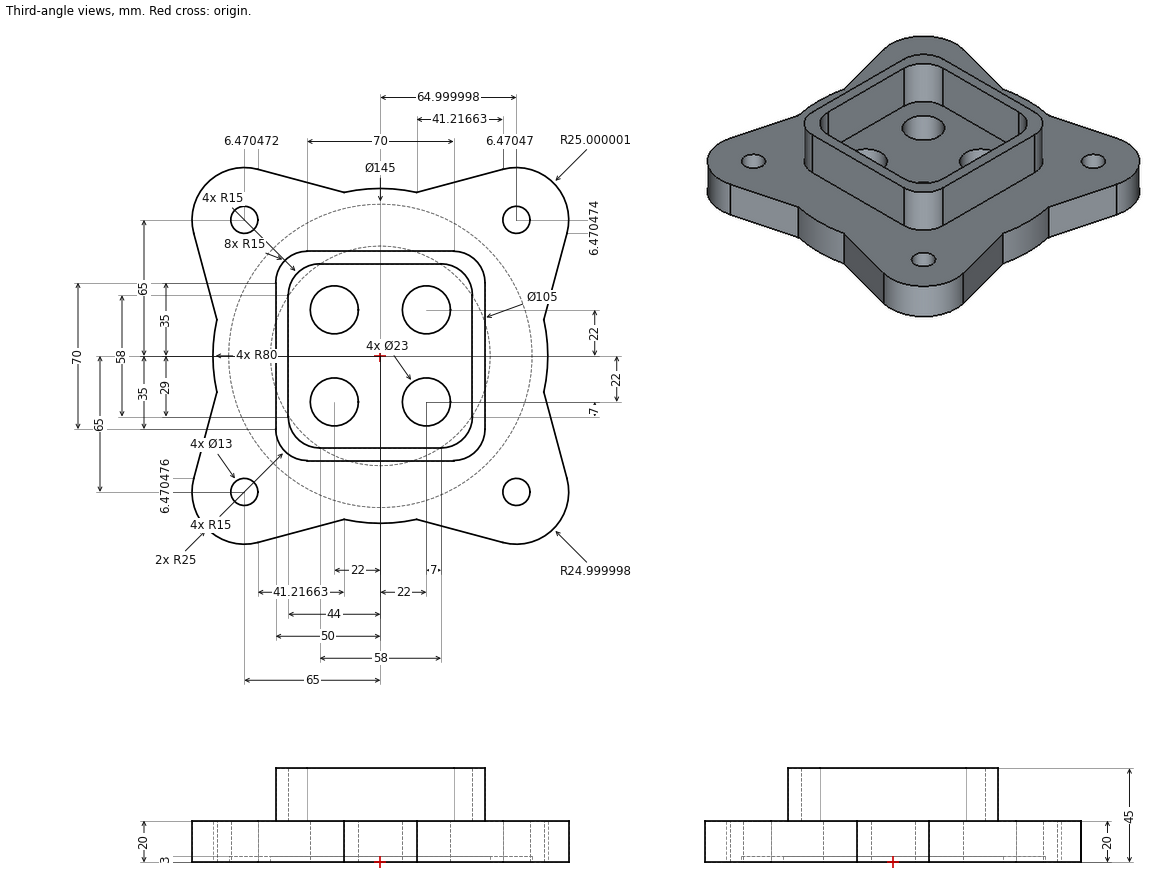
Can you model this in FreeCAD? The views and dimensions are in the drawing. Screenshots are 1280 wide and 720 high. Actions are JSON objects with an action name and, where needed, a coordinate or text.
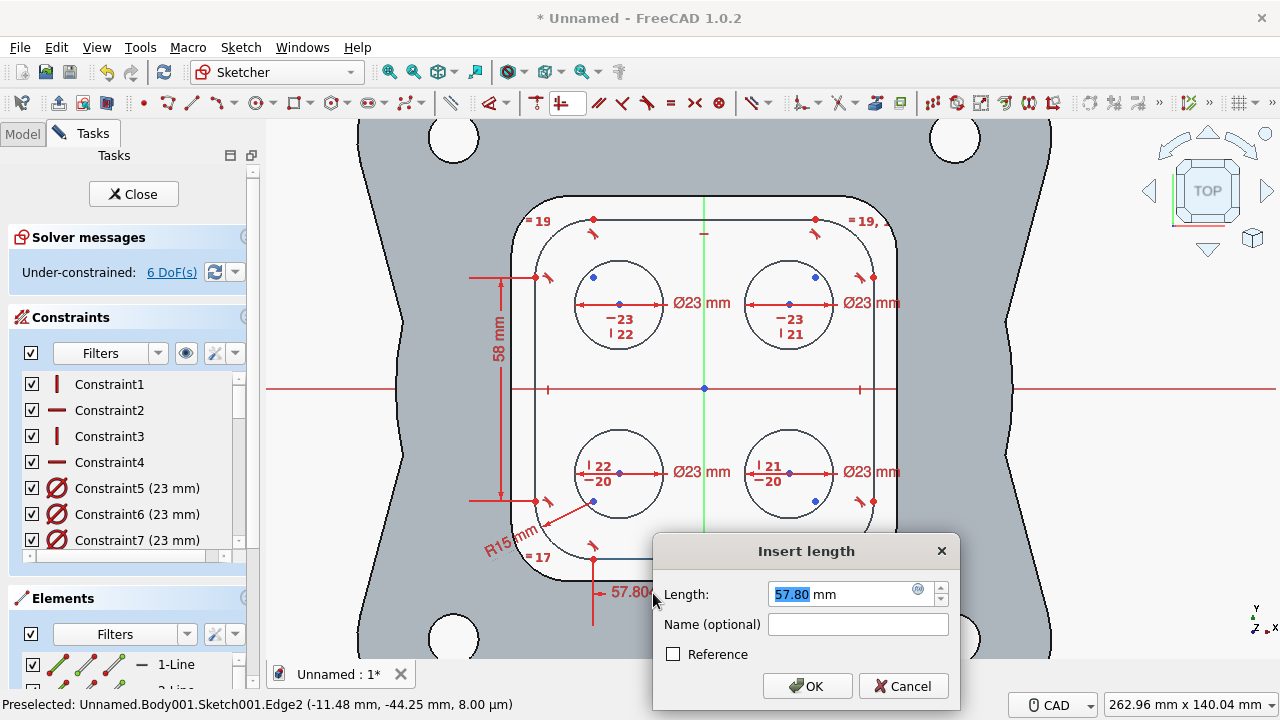
{"action": "type", "text": "58"}
{"action": "key", "text": "Return"}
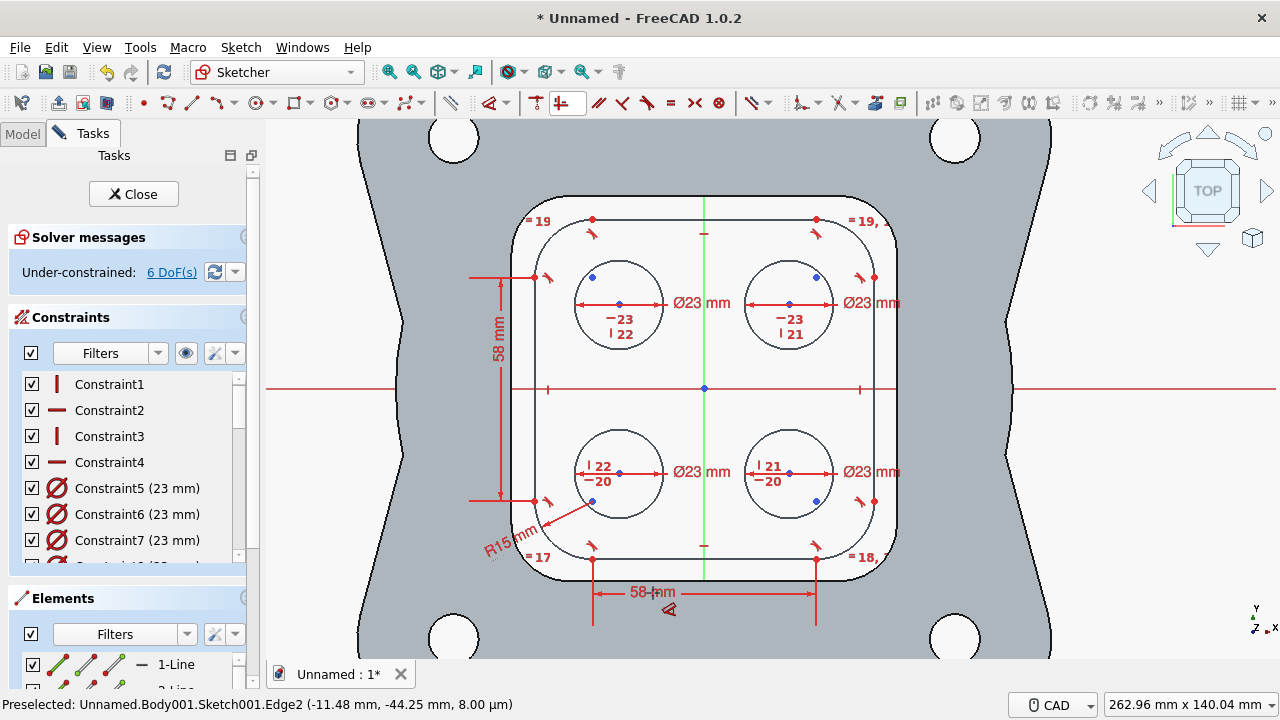
{"action": "left_click", "coordinate": [789, 474]}
{"action": "left_click", "coordinate": [727, 508]}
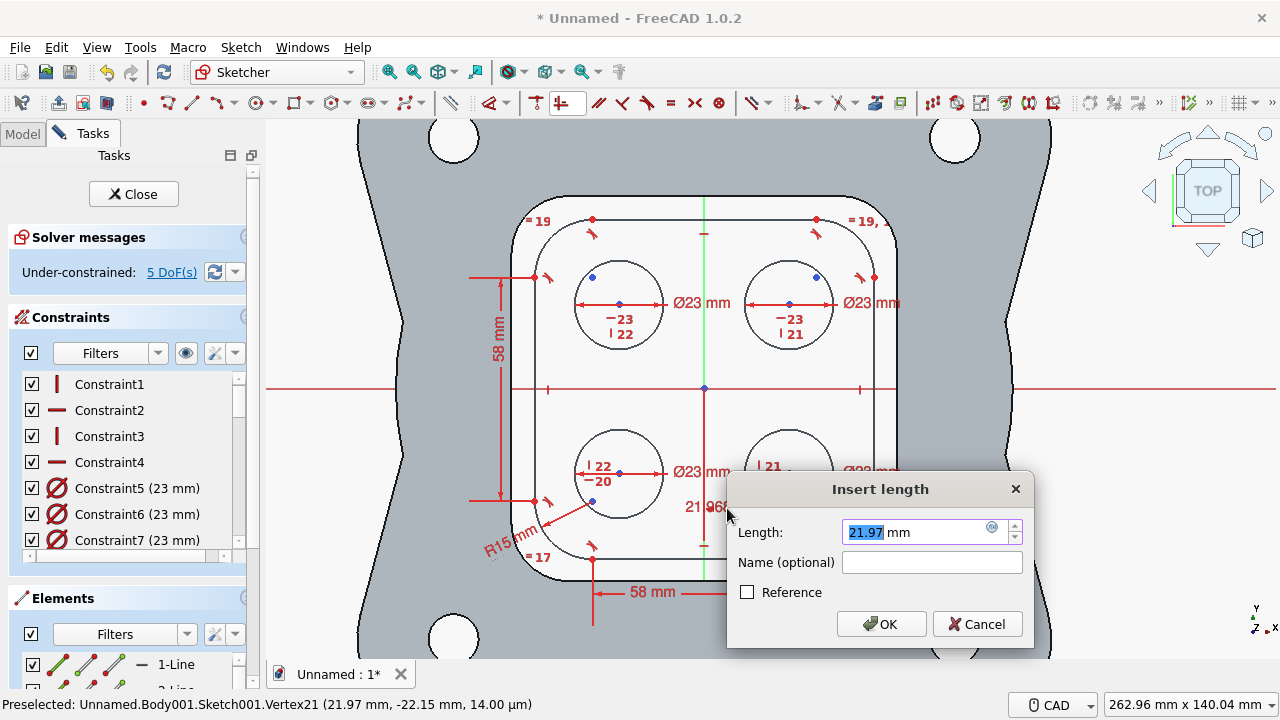
{"action": "type", "text": "22"}
{"action": "key", "text": "Return"}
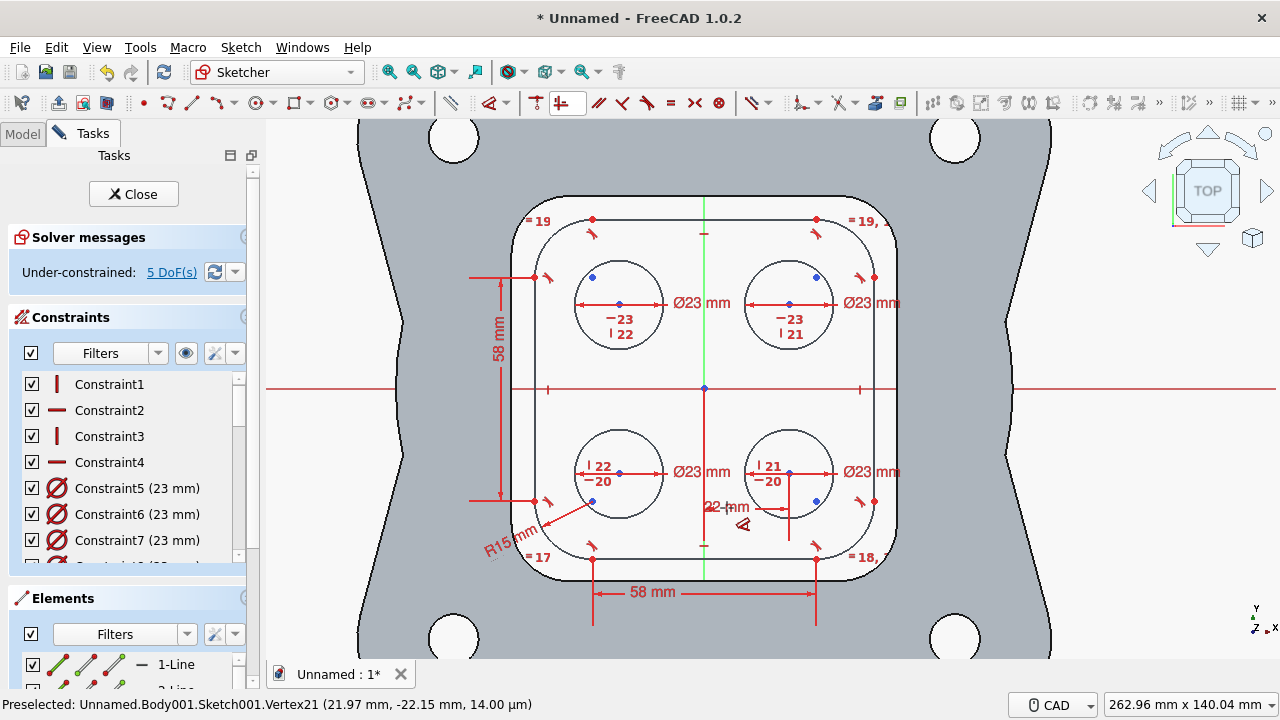
{"action": "left_click", "coordinate": [789, 474]}
{"action": "left_click", "coordinate": [823, 412]}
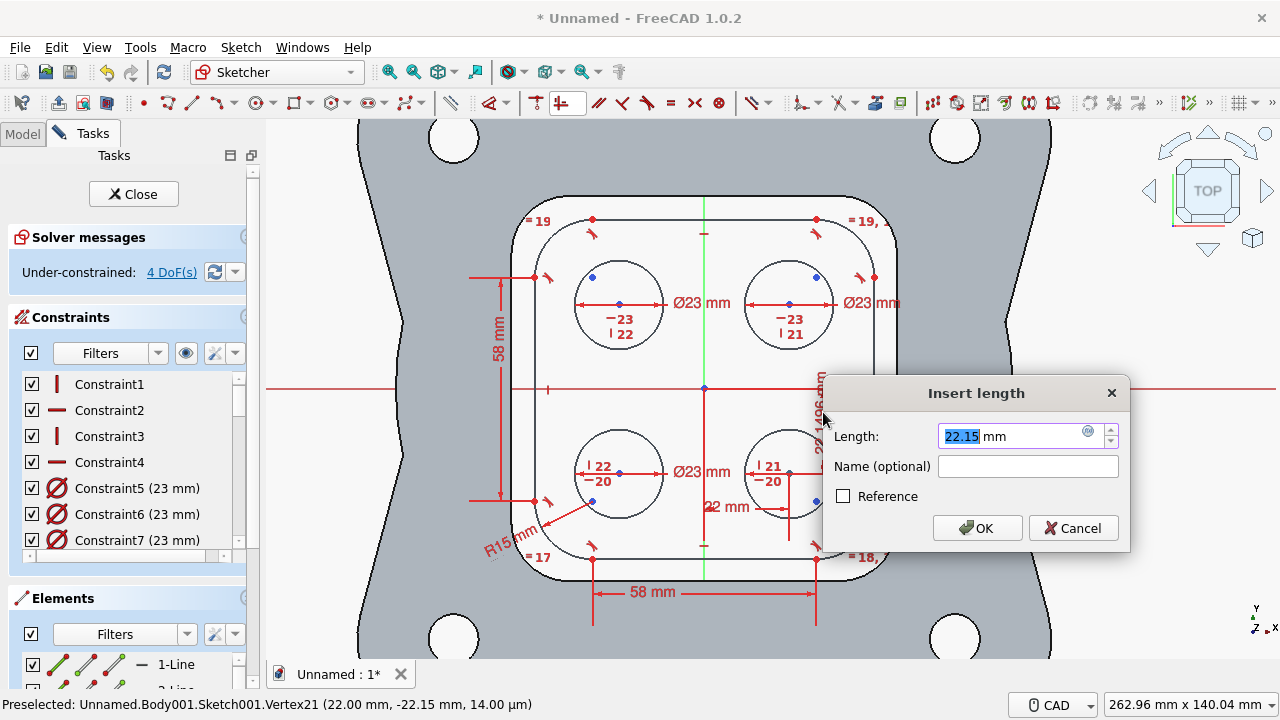
{"action": "type", "text": "22"}
{"action": "key", "text": "Return"}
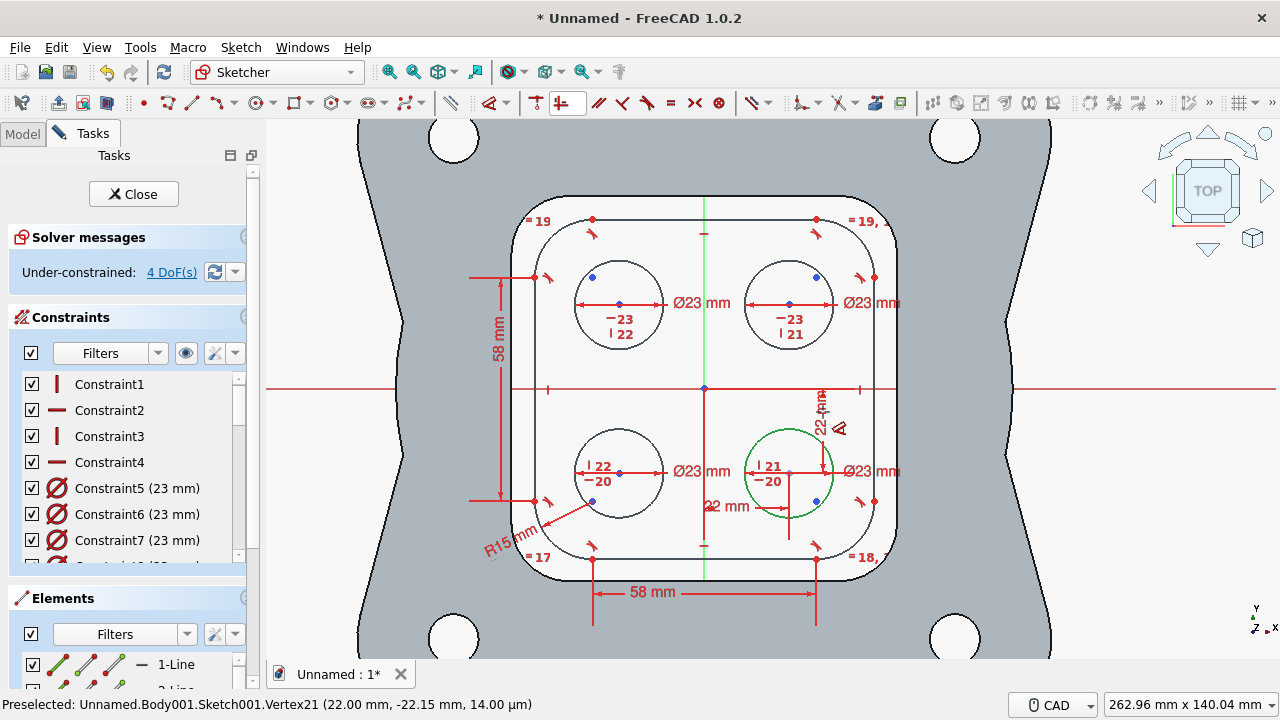
{"action": "left_click", "coordinate": [619, 473]}
{"action": "left_click", "coordinate": [662, 355]}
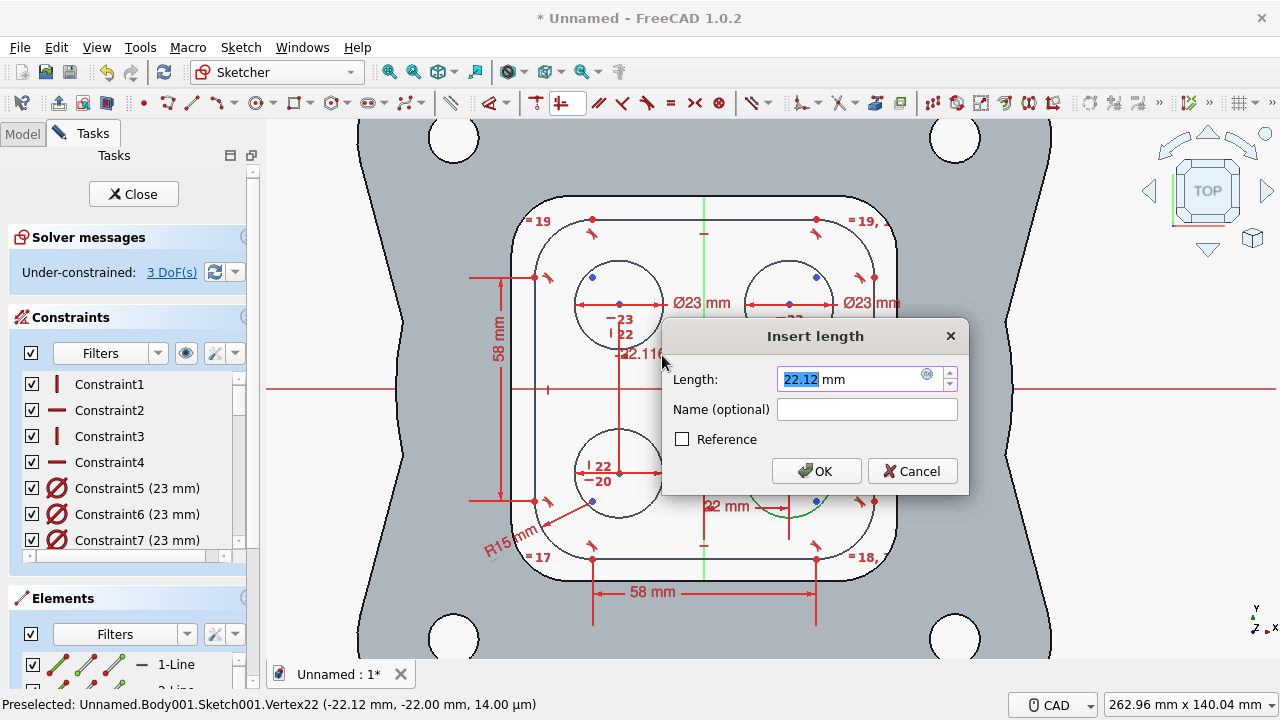
{"action": "type", "text": "22"}
{"action": "key", "text": "Return"}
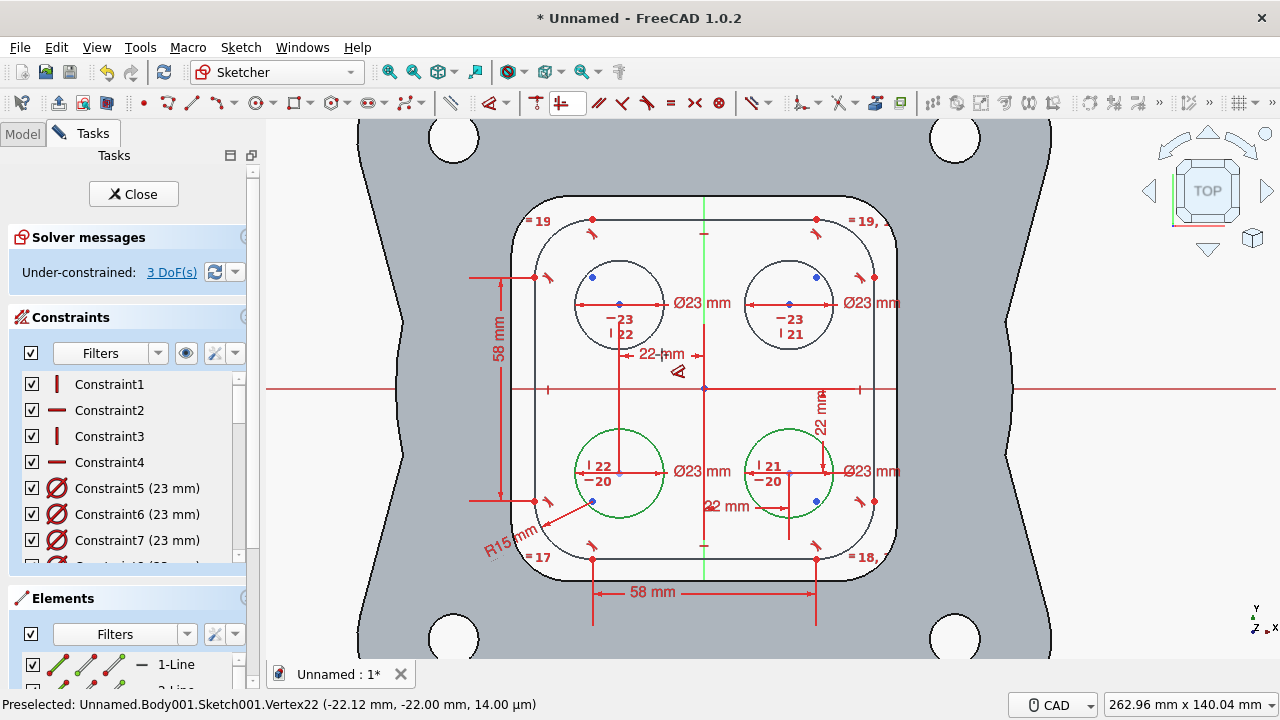
{"action": "left_click", "coordinate": [789, 305]}
{"action": "left_click", "coordinate": [823, 366]}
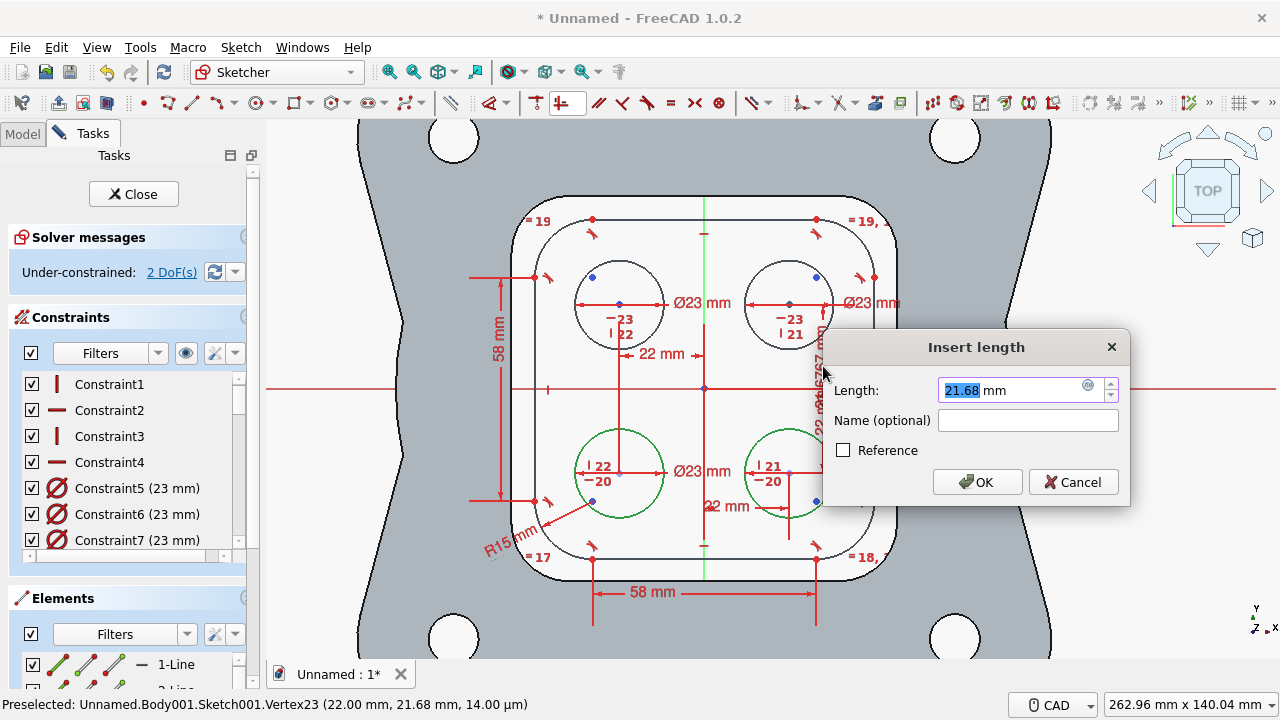
{"action": "type", "text": "22"}
{"action": "key", "text": "Return"}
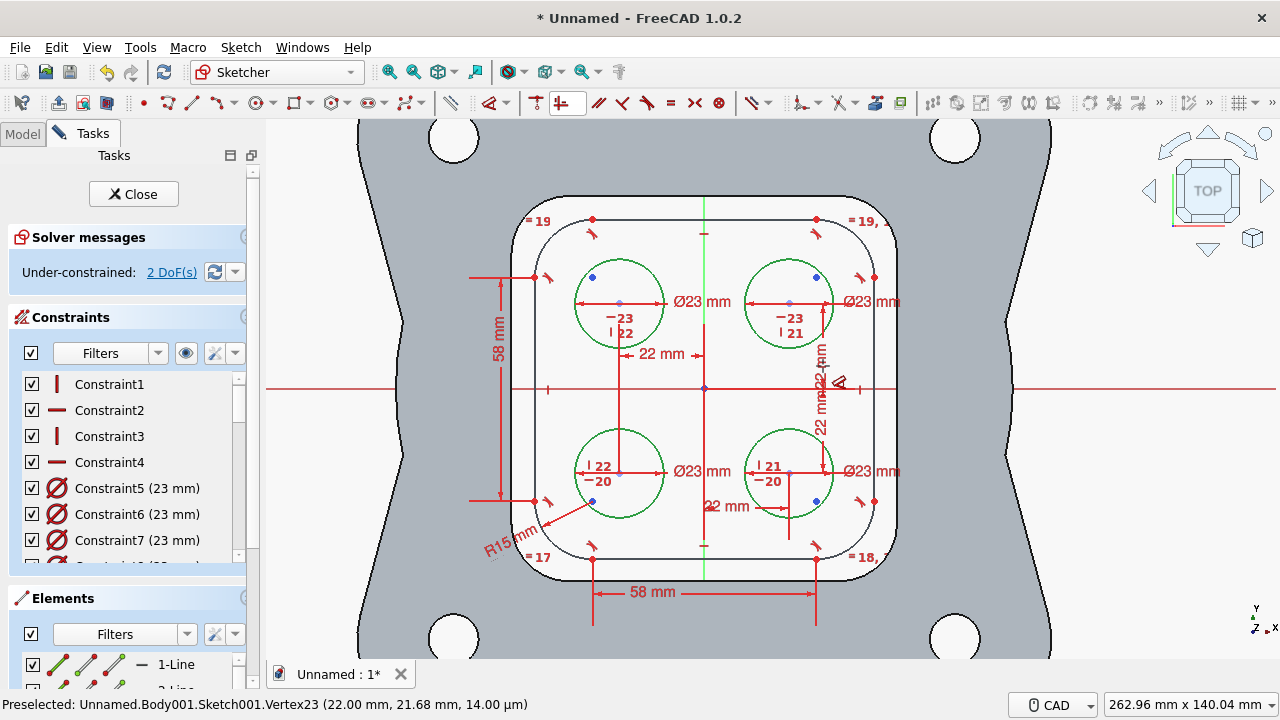
{"action": "scroll", "coordinate": [816, 559], "scroll_direction": "up", "scroll_amount": 2}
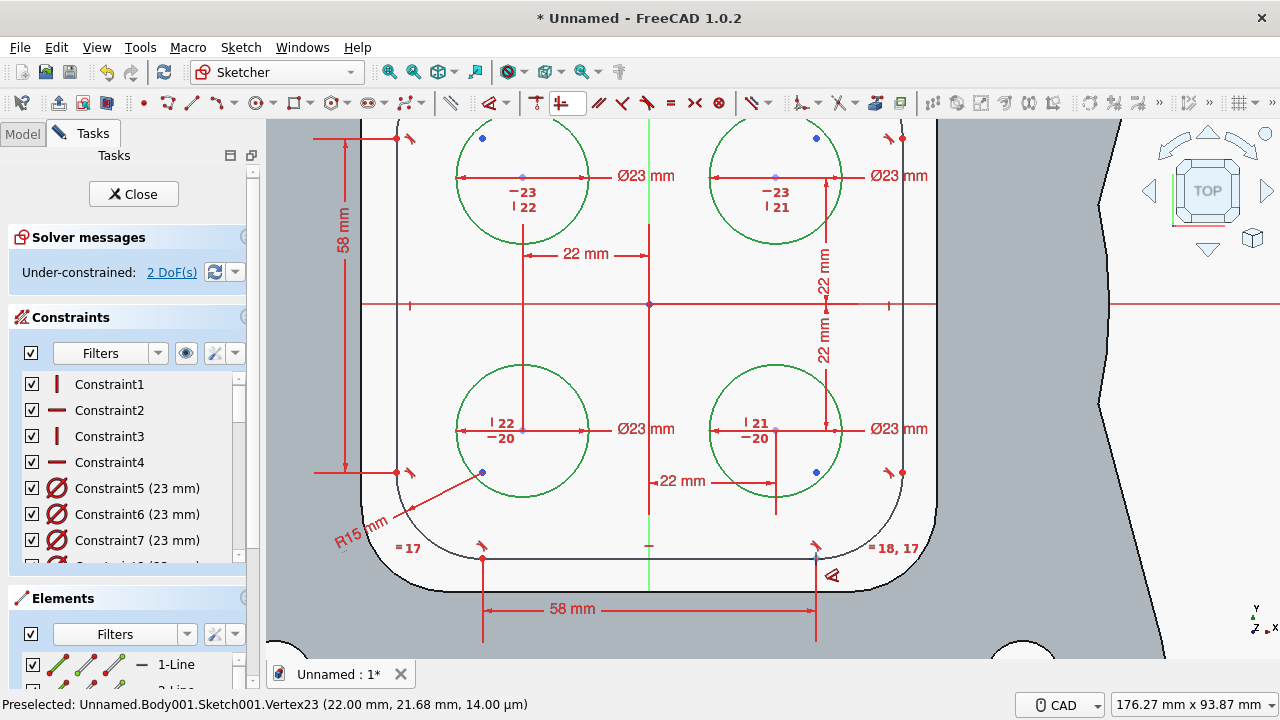
{"action": "left_click", "coordinate": [816, 559]}